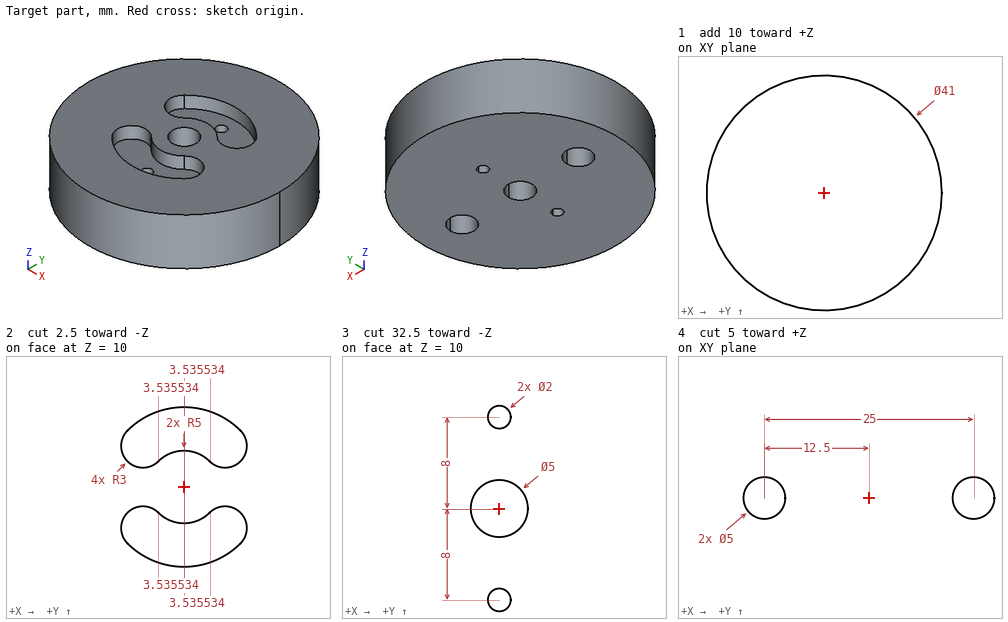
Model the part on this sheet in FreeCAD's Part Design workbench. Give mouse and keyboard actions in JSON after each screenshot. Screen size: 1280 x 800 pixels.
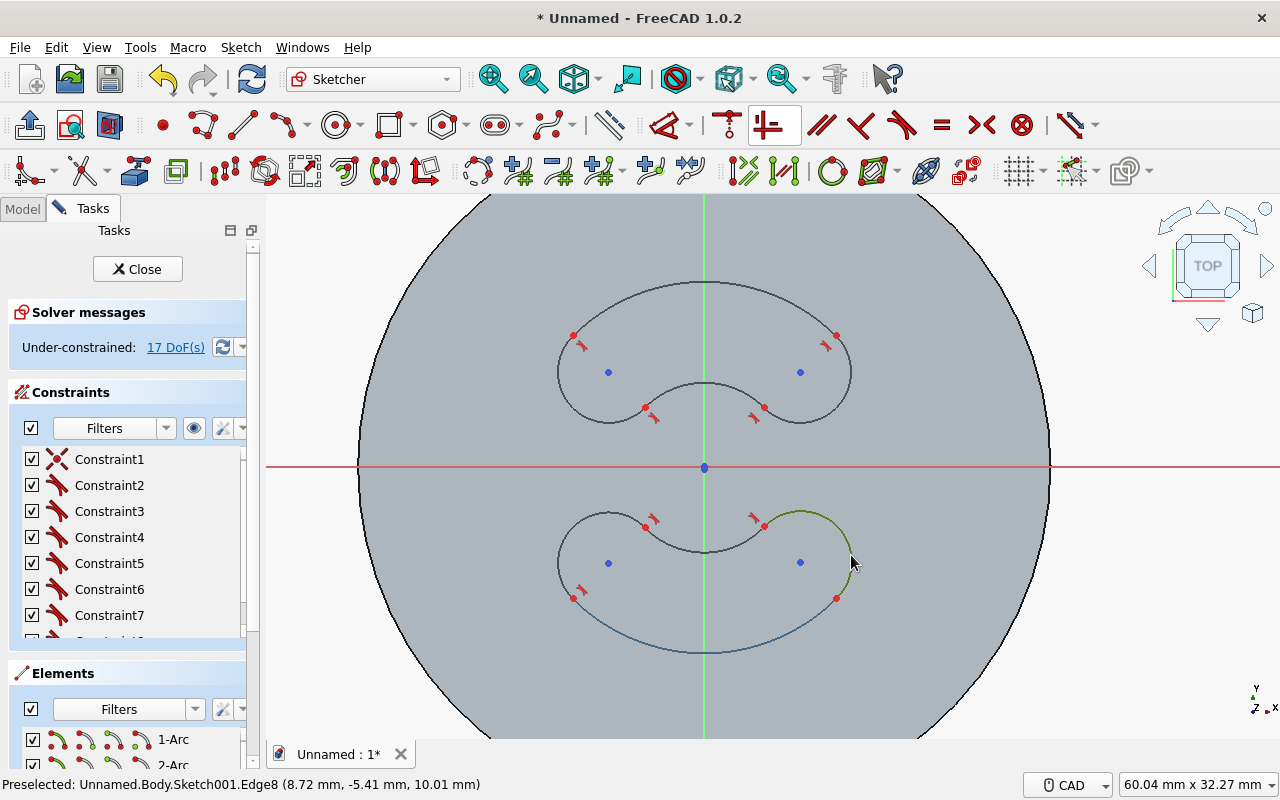
{"action": "key", "text": "t"}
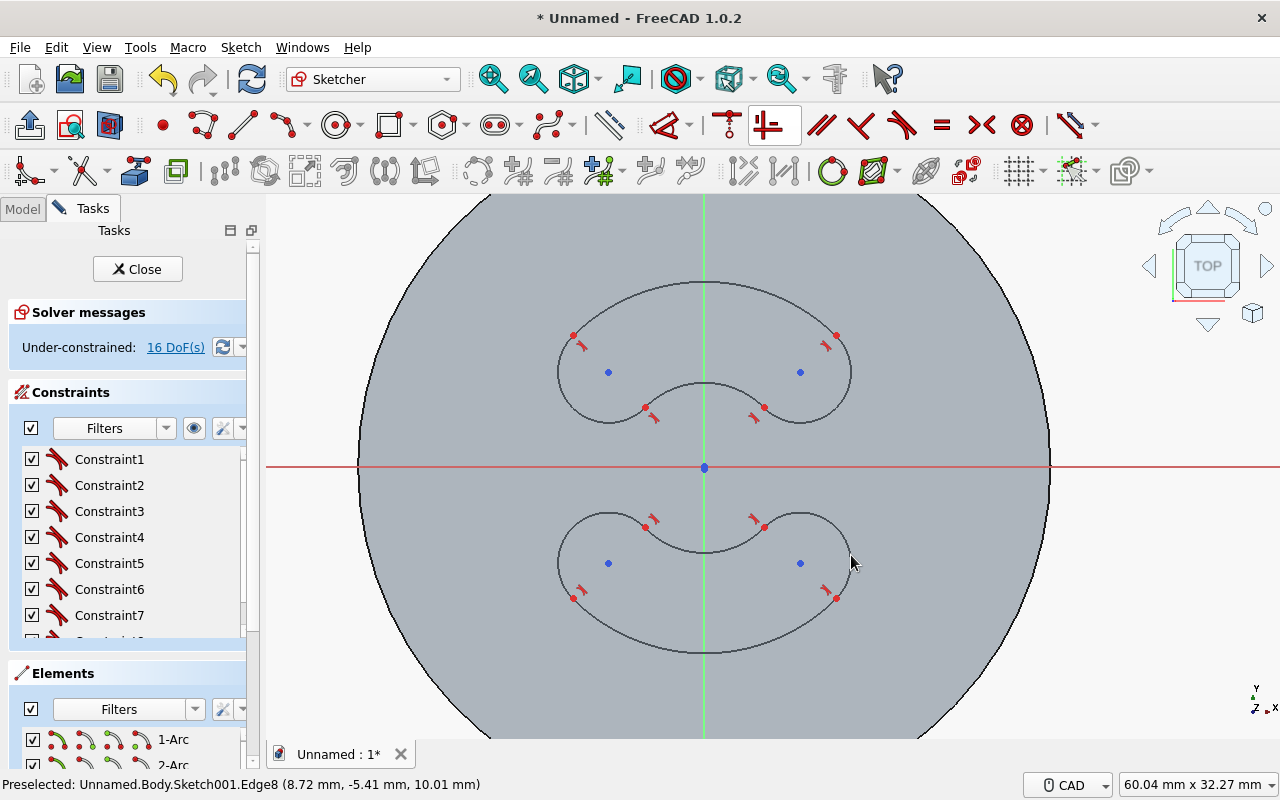
{"action": "left_click", "coordinate": [731, 387]}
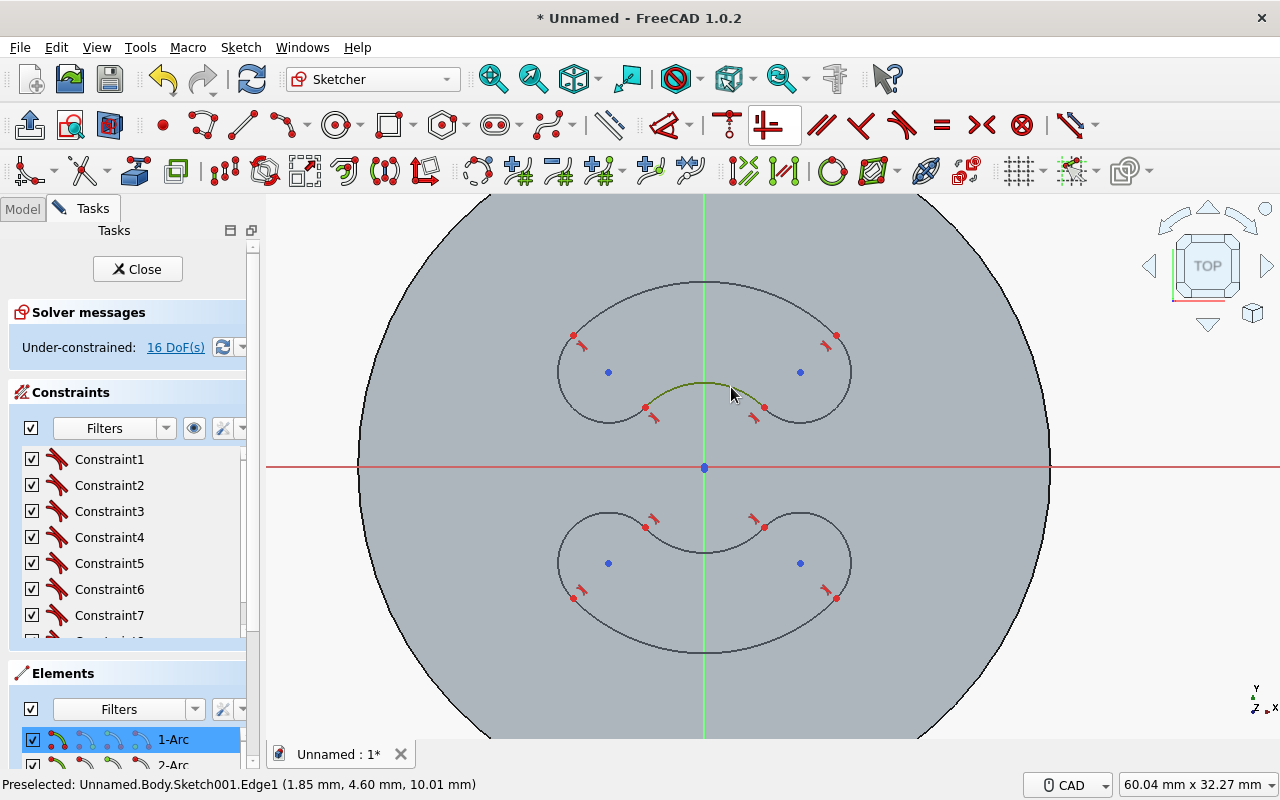
{"action": "left_click", "coordinate": [762, 291]}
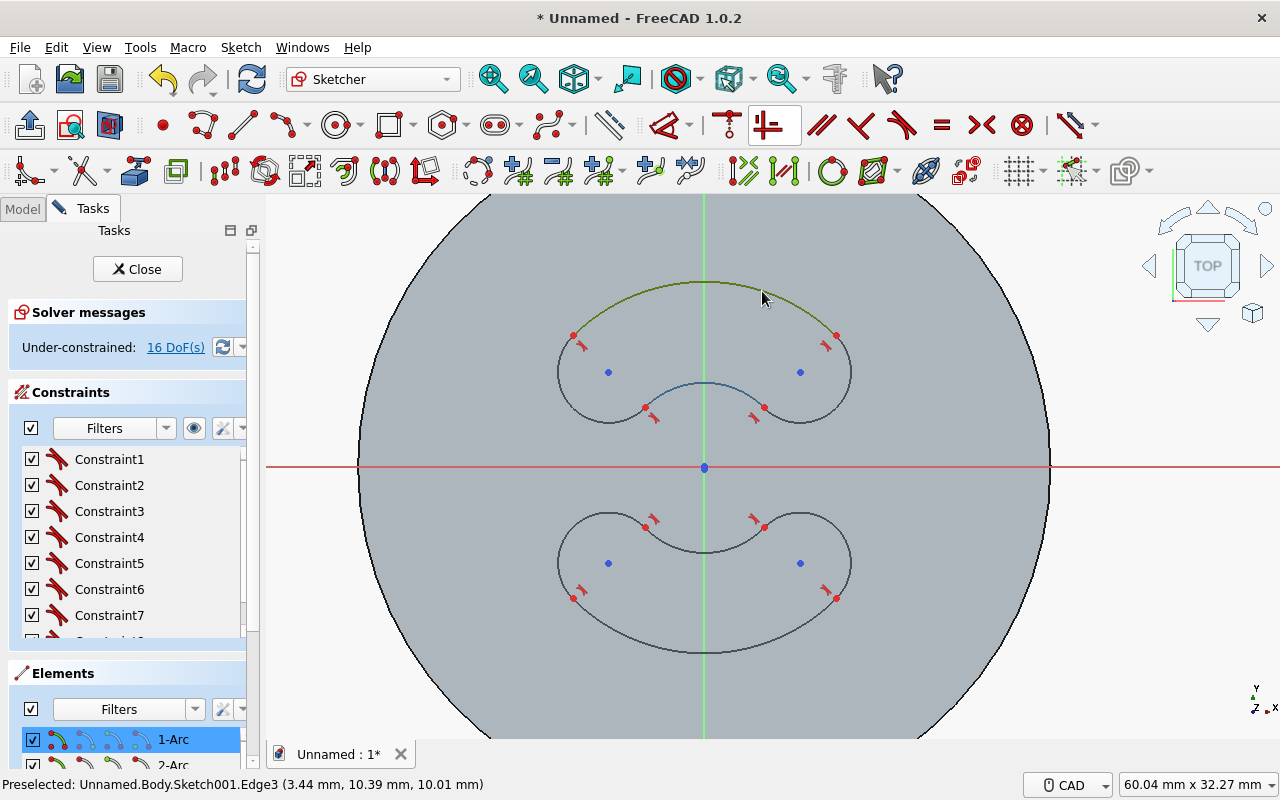
{"action": "key", "text": "c"}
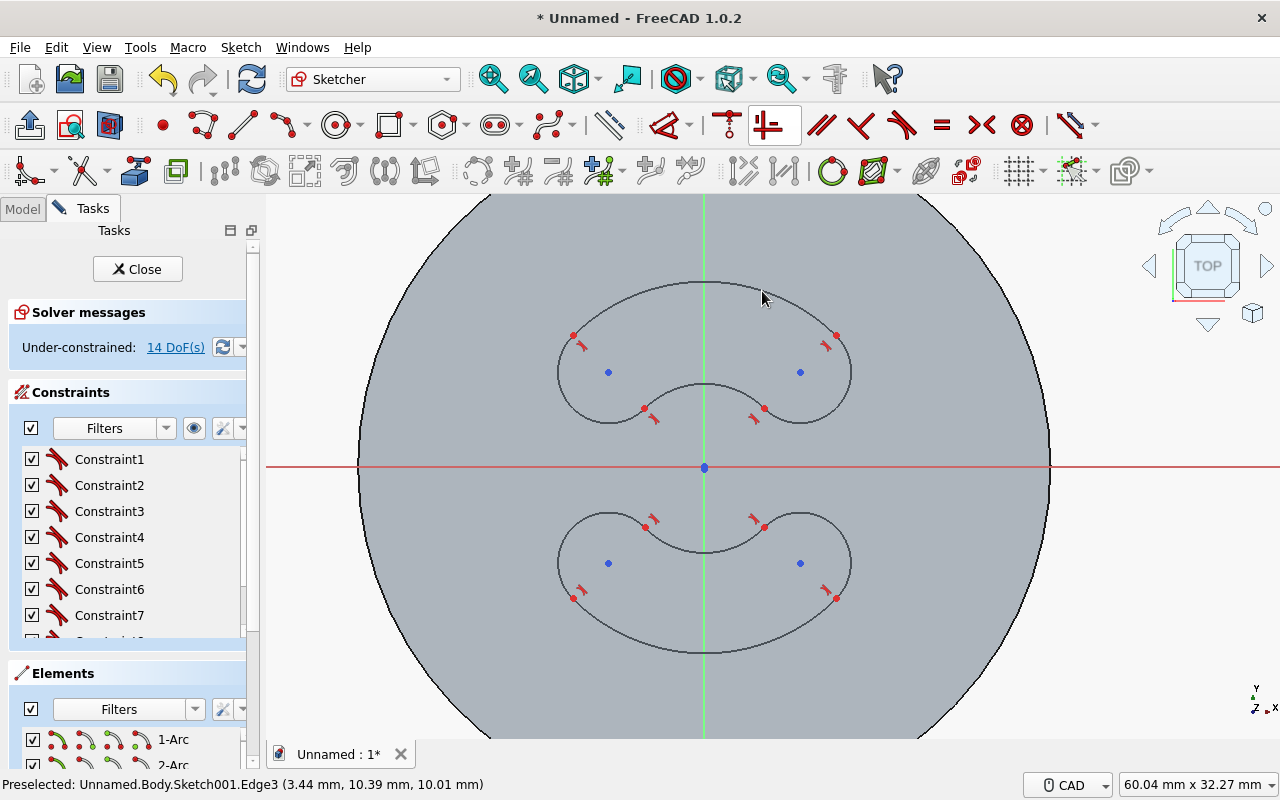
{"action": "left_click", "coordinate": [731, 388]}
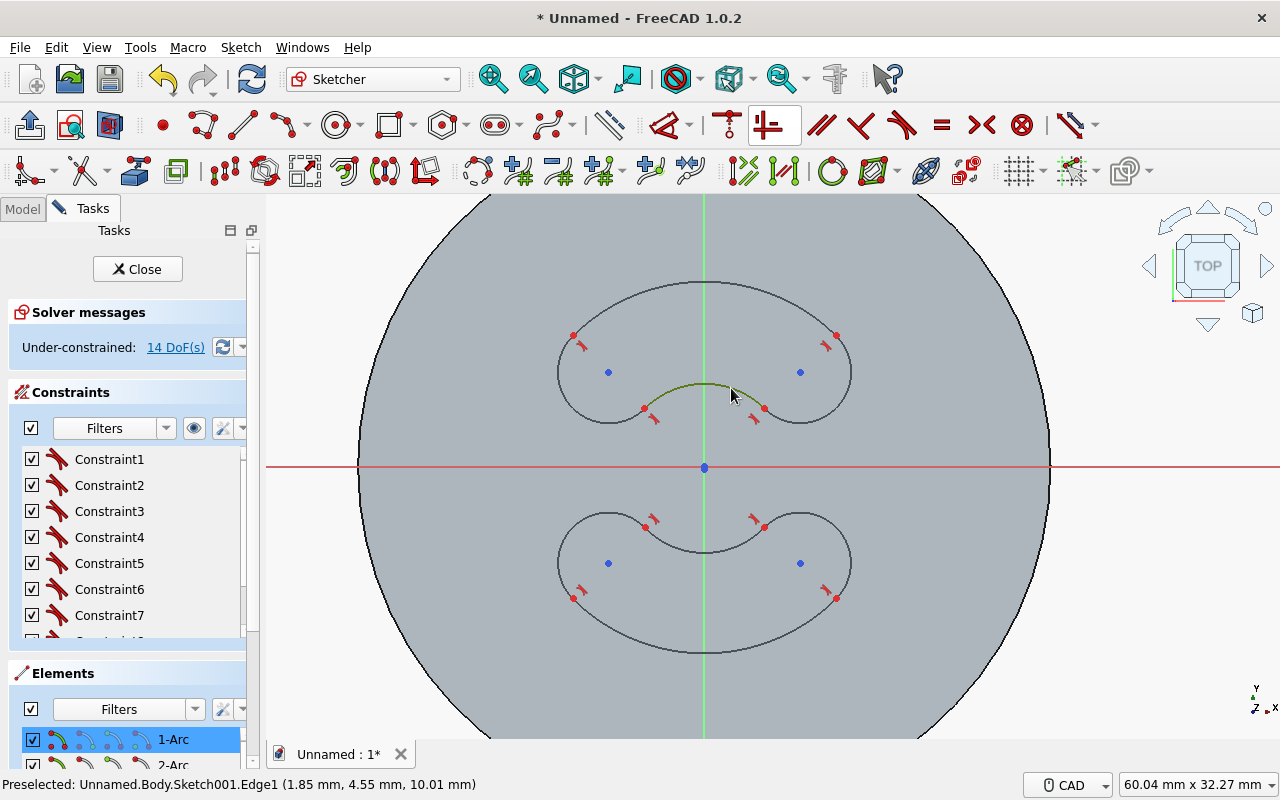
{"action": "left_click", "coordinate": [678, 549]}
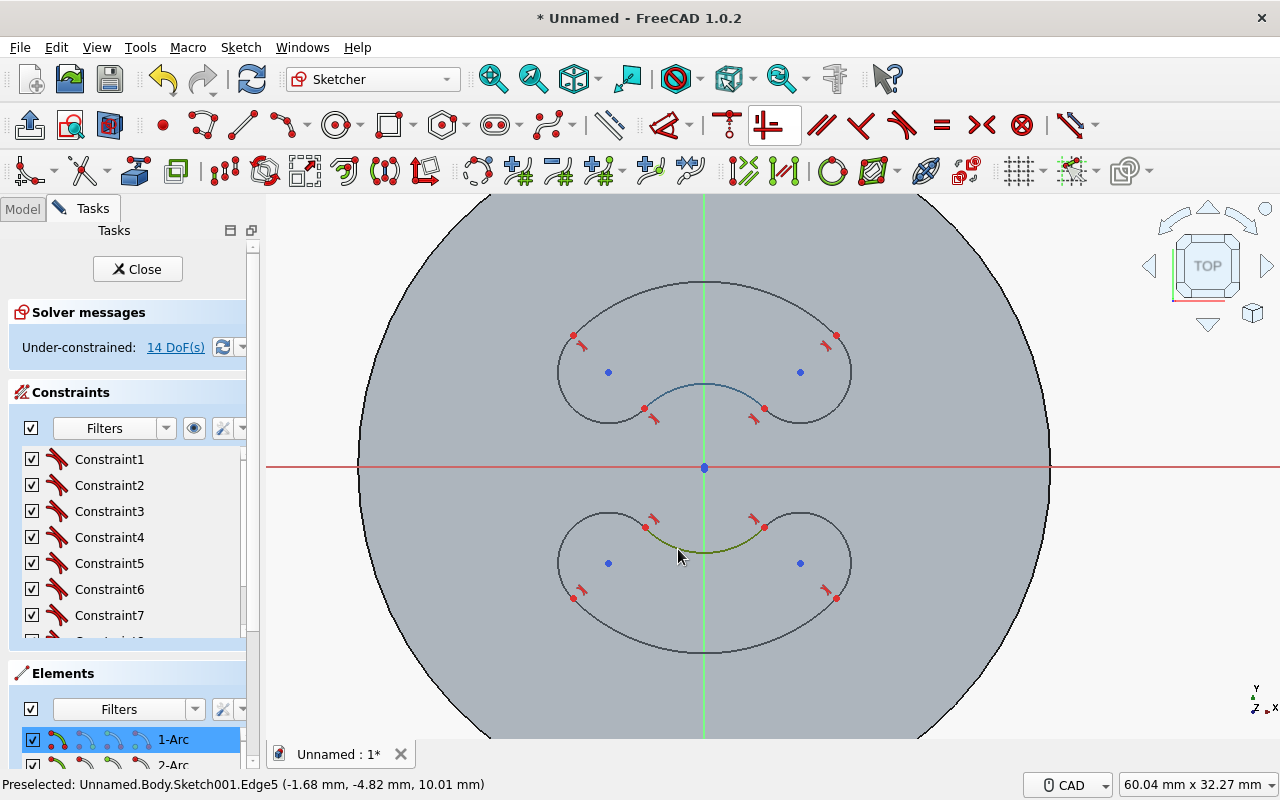
{"action": "key", "text": "c"}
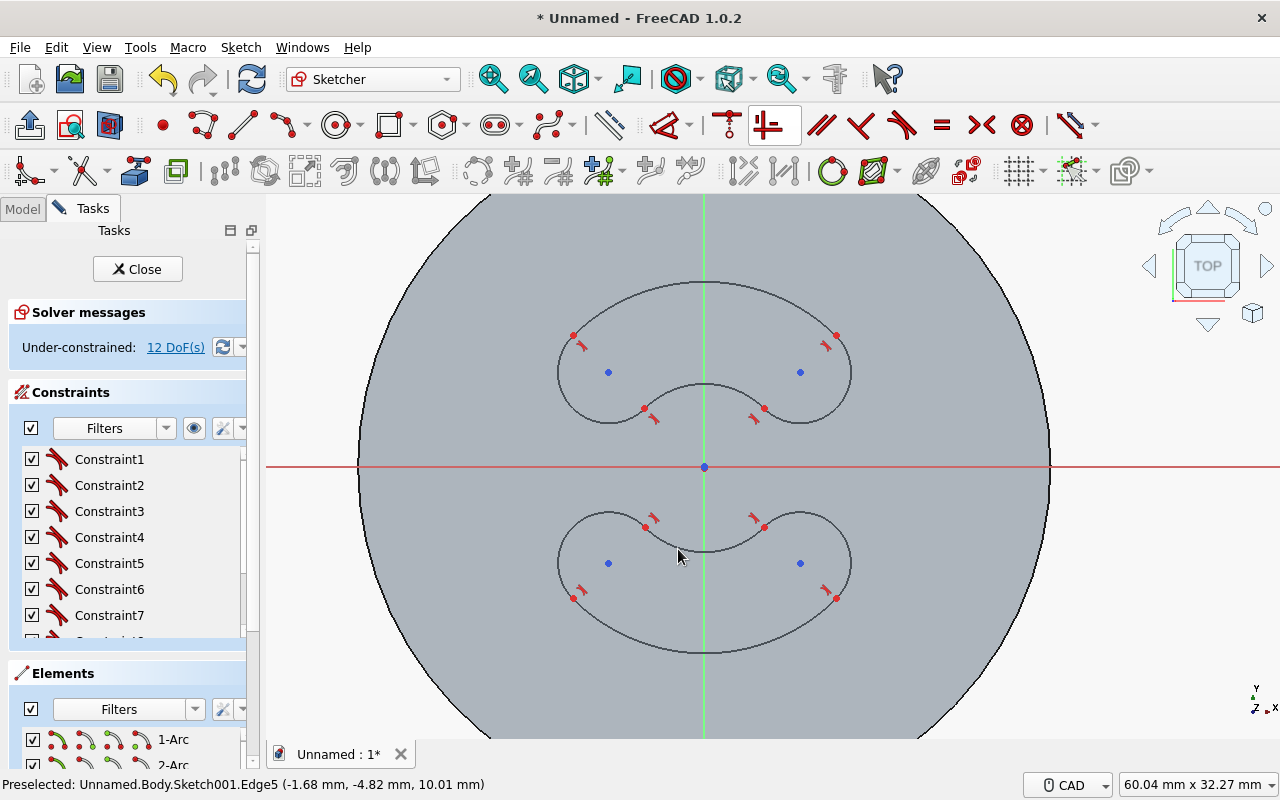
{"action": "left_click", "coordinate": [731, 388]}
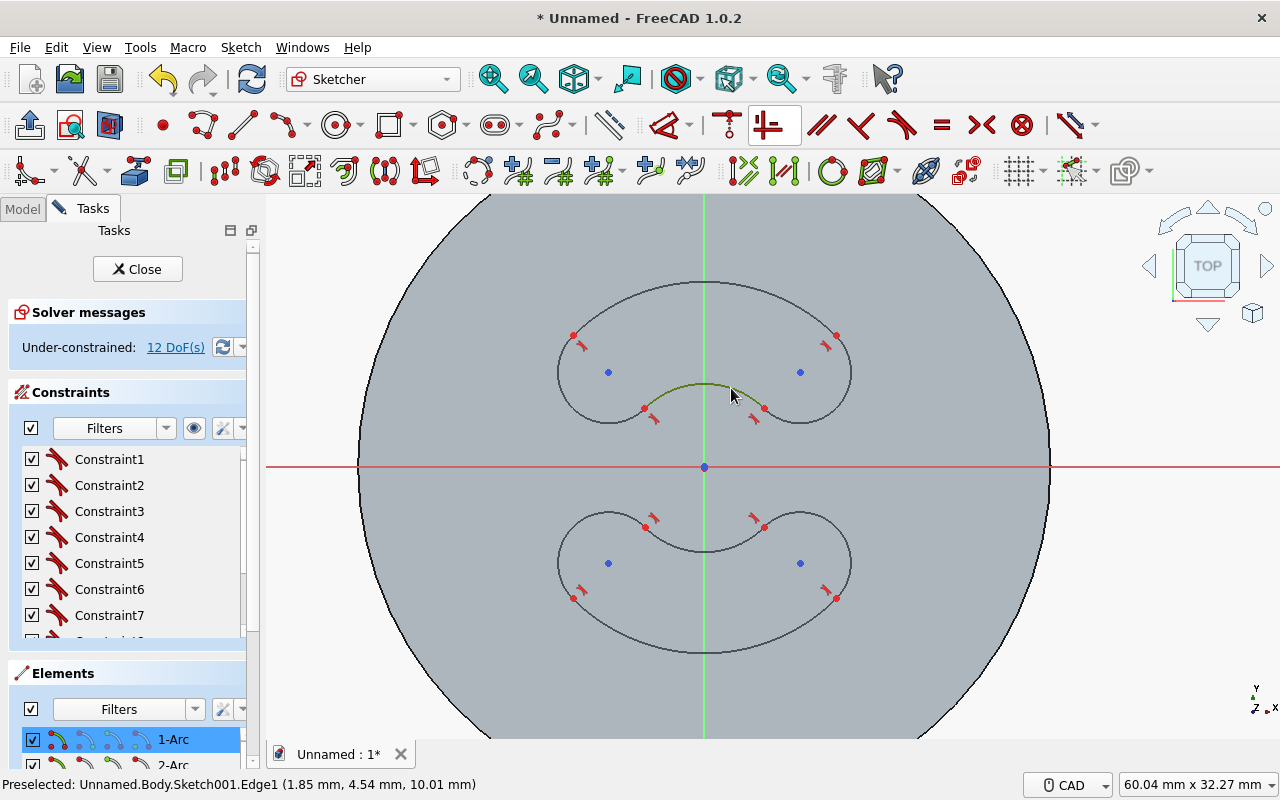
{"action": "left_click", "coordinate": [647, 644]}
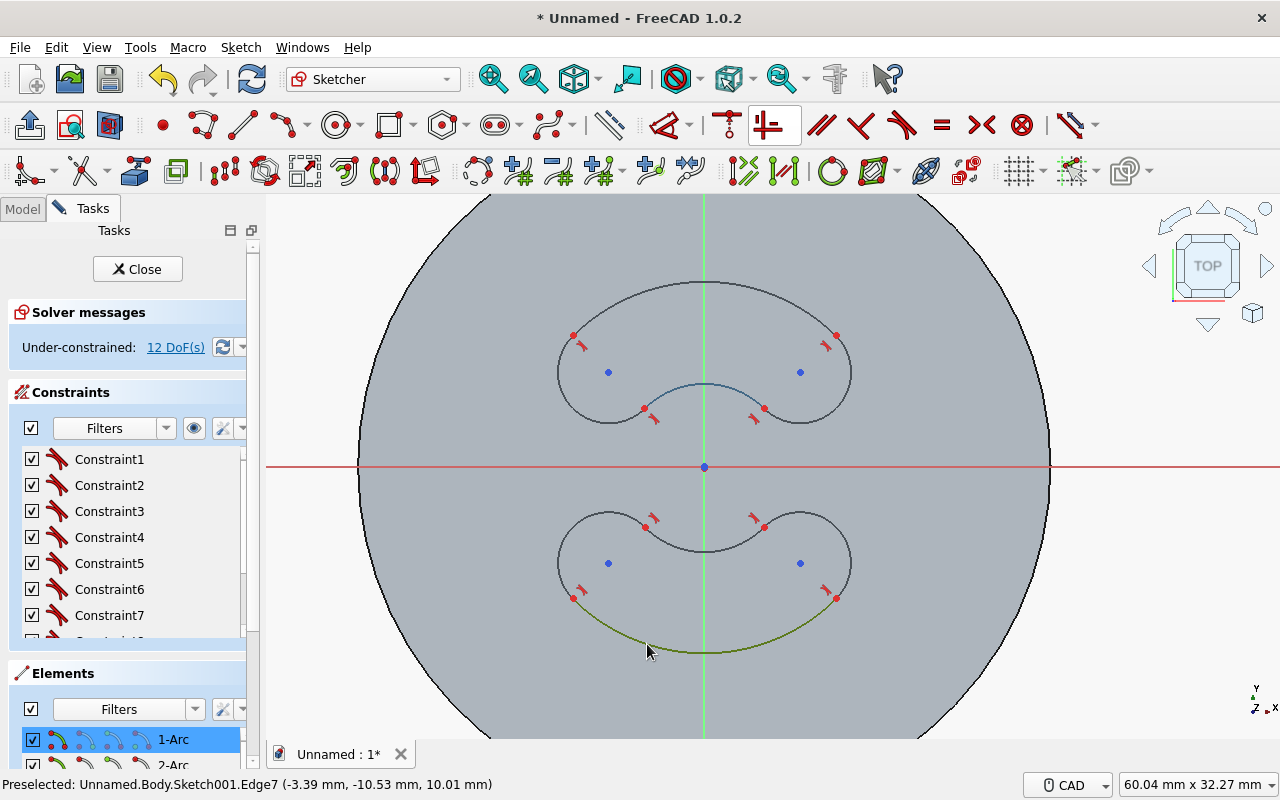
{"action": "key", "text": "c"}